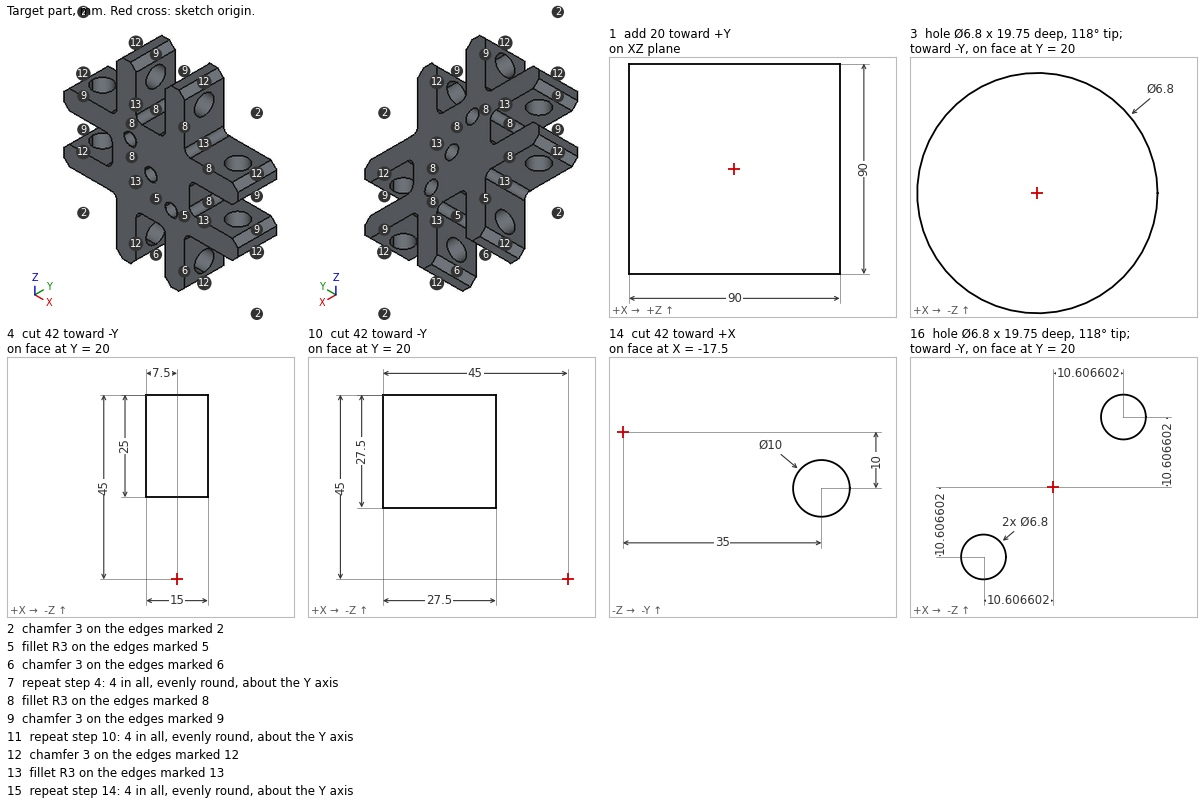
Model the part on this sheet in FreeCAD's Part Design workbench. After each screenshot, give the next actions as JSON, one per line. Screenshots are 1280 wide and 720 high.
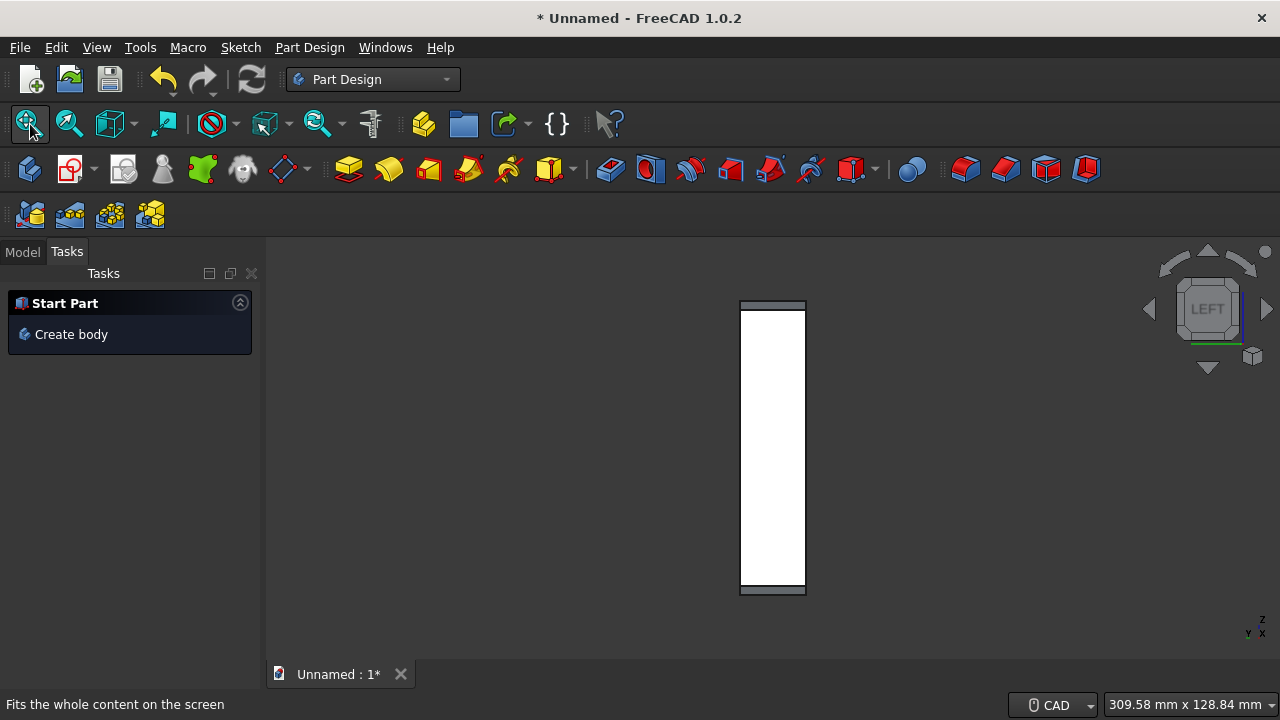
{"action": "key", "text": "v 3"}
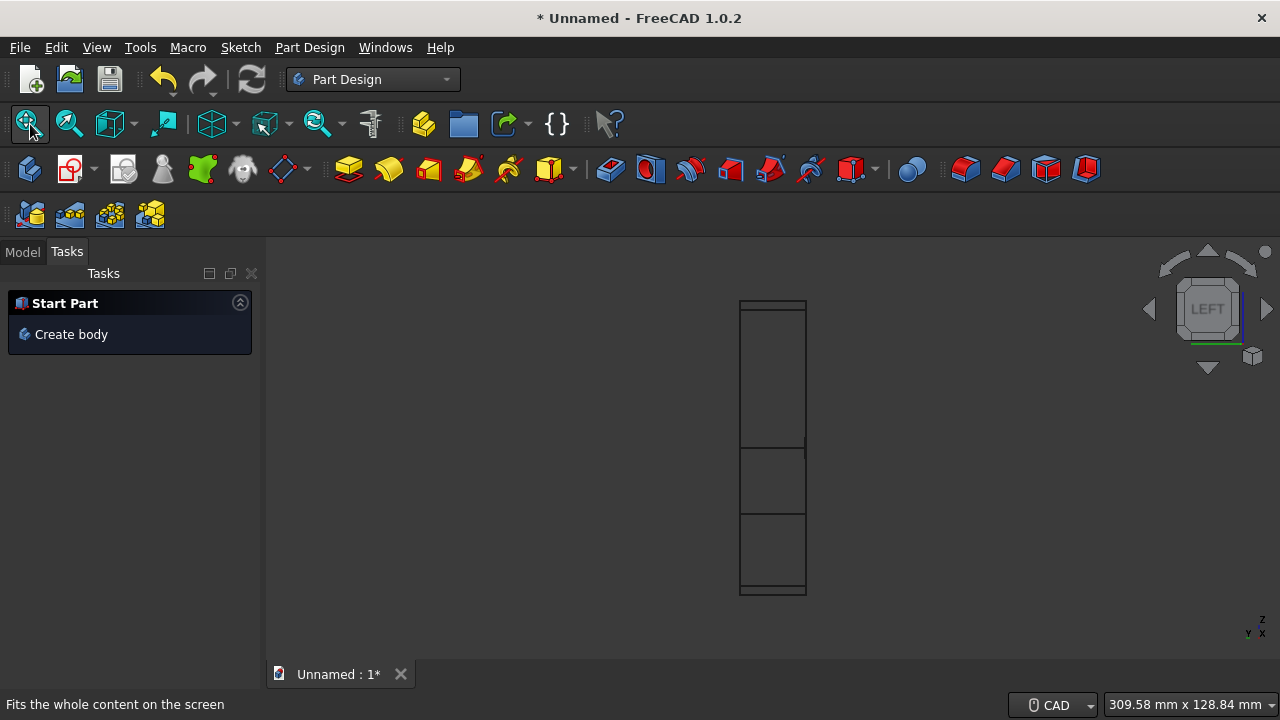
{"action": "key", "text": "0"}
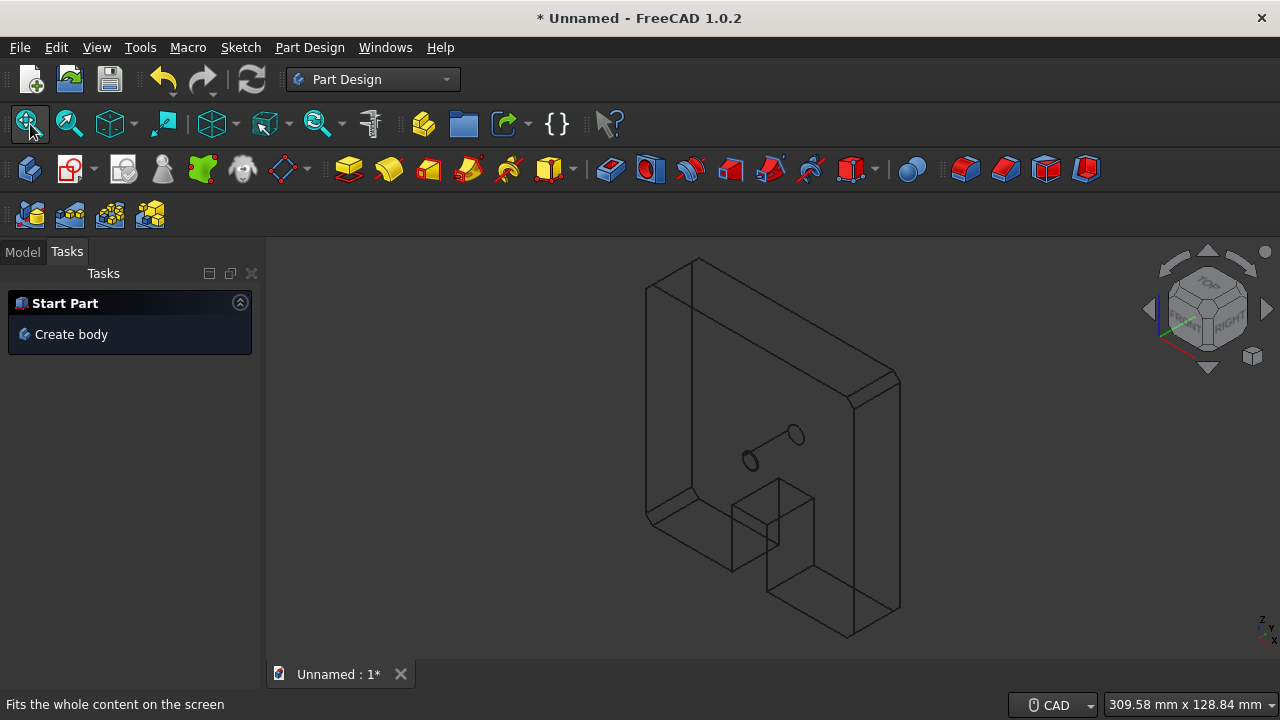
{"action": "left_click", "coordinate": [790, 511]}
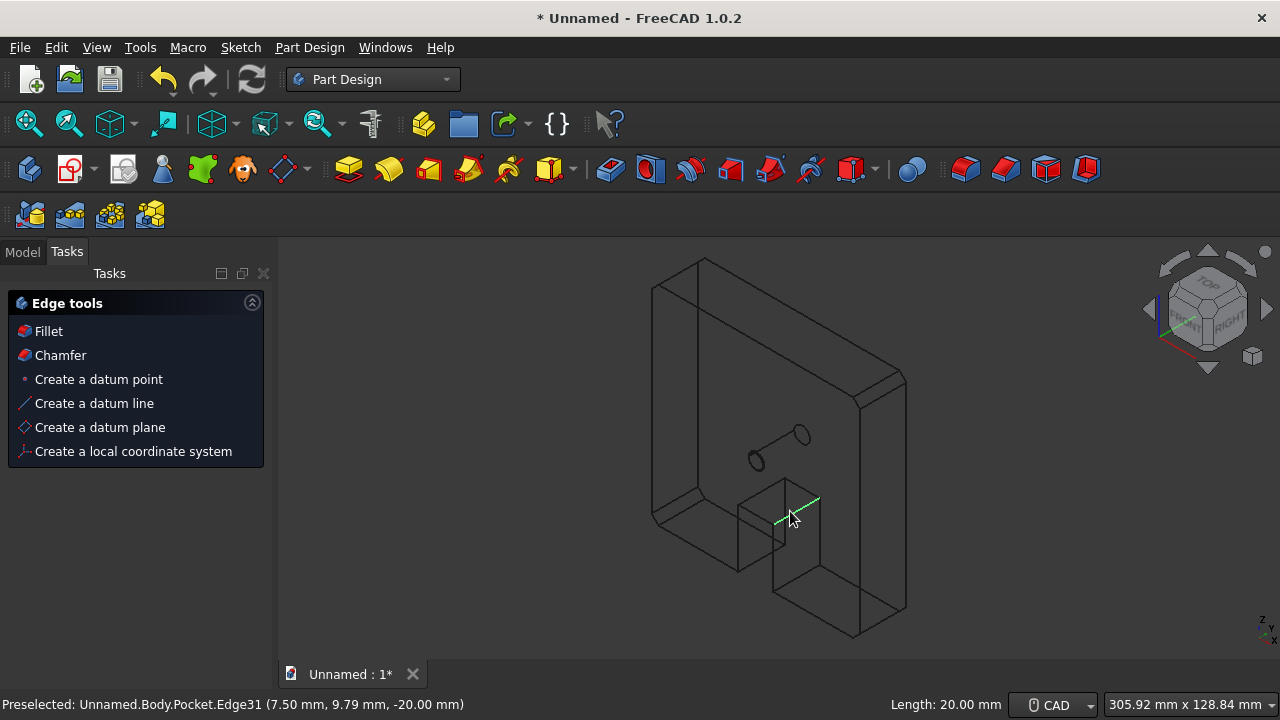
{"action": "left_click", "coordinate": [762, 490], "text": "ctrl"}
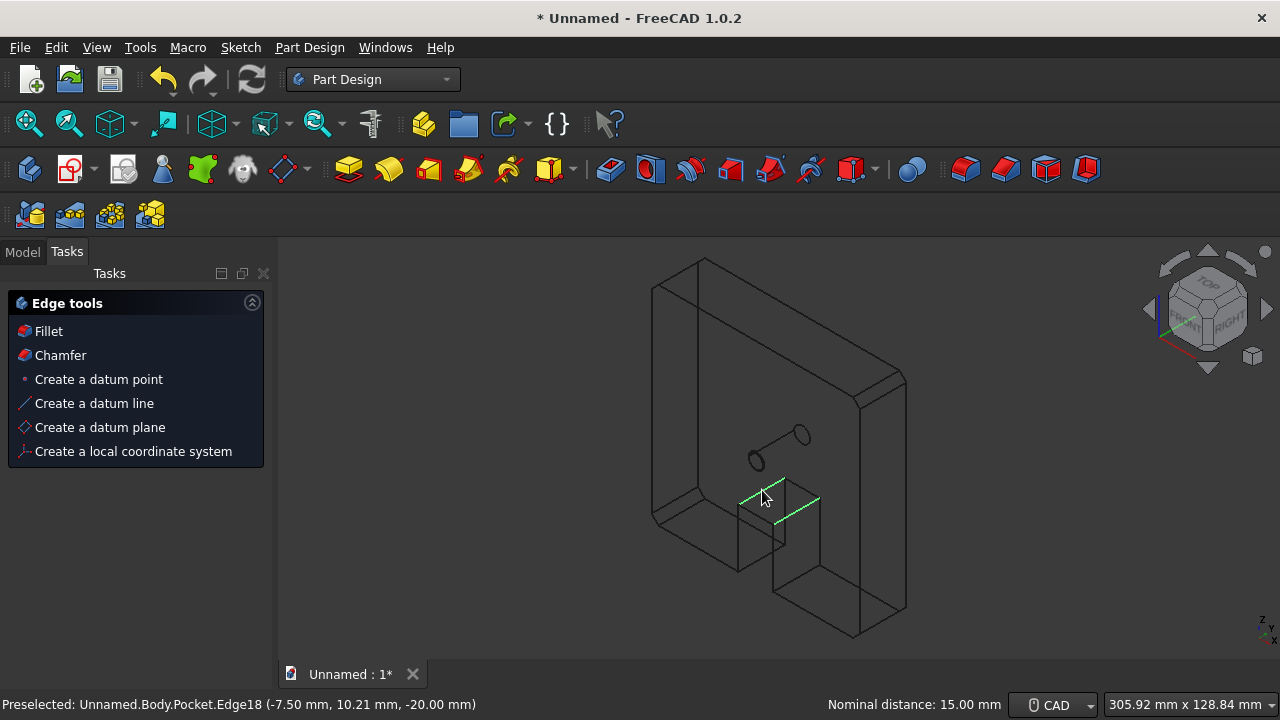
{"action": "key", "text": "v 1"}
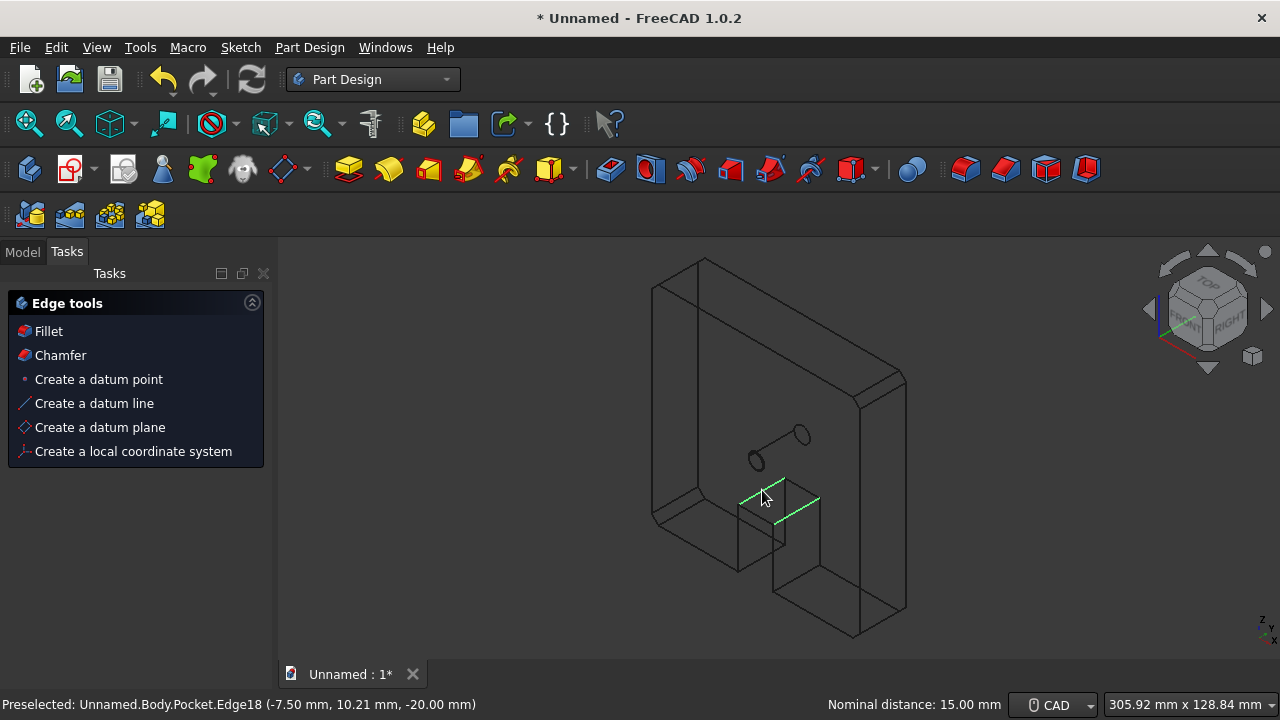
{"action": "left_click", "coordinate": [966, 170]}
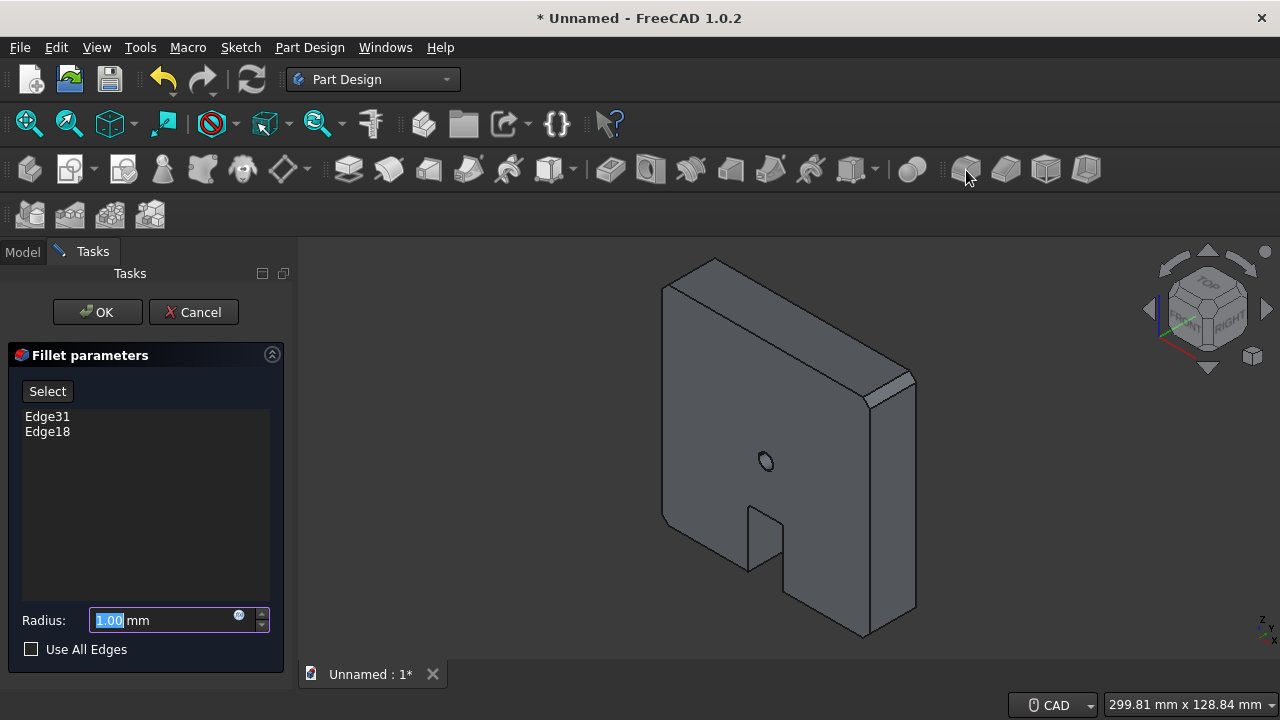
{"action": "type", "text": "3"}
{"action": "key", "text": "Tab"}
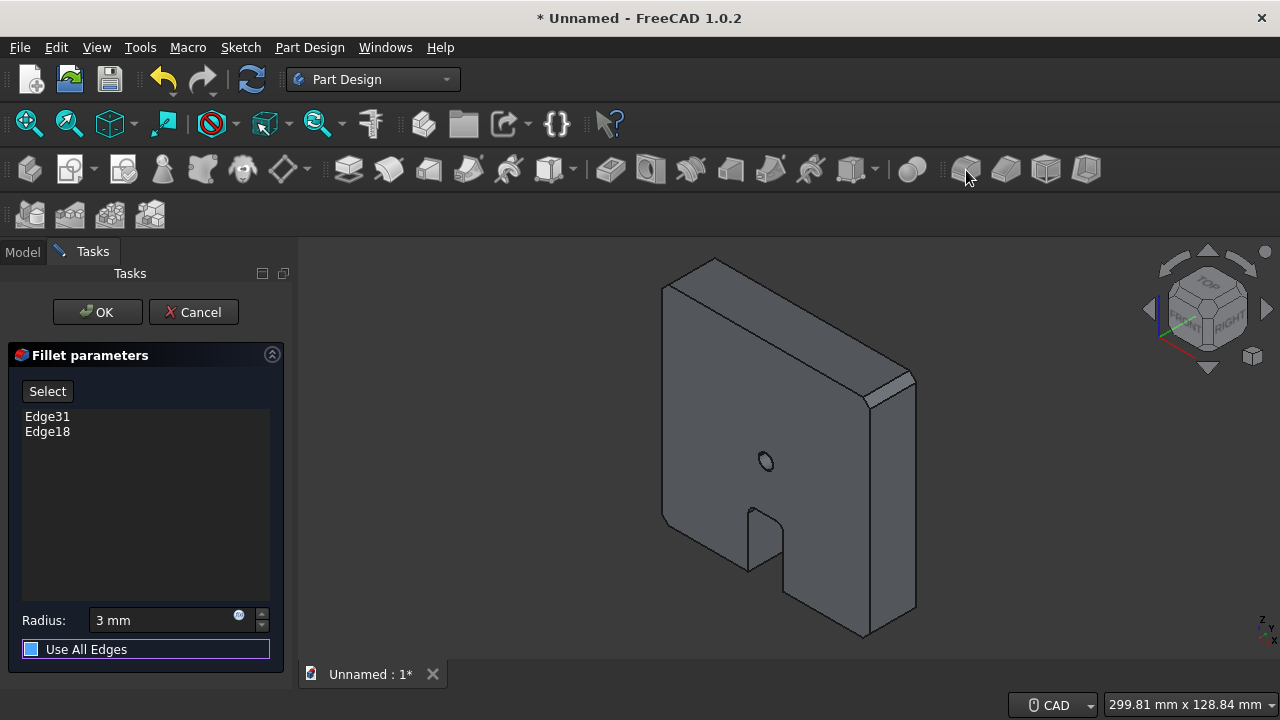
{"action": "left_click", "coordinate": [98, 312]}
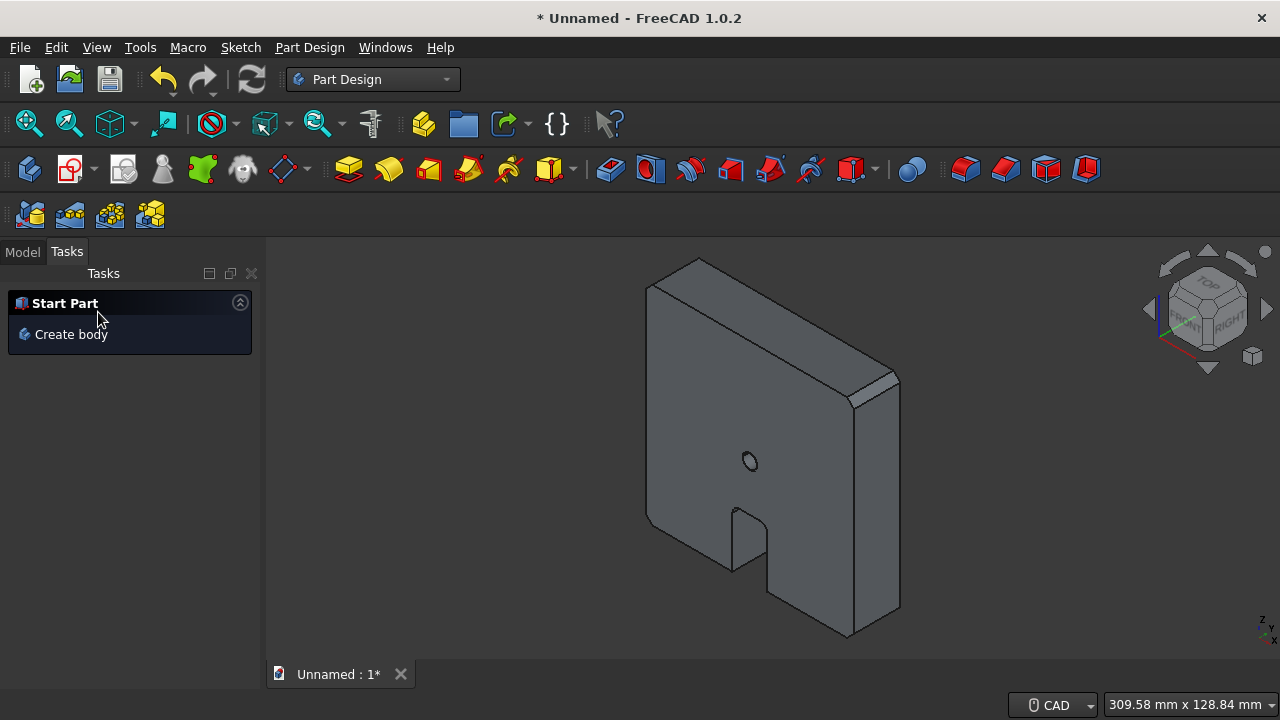
{"action": "key", "text": "2"}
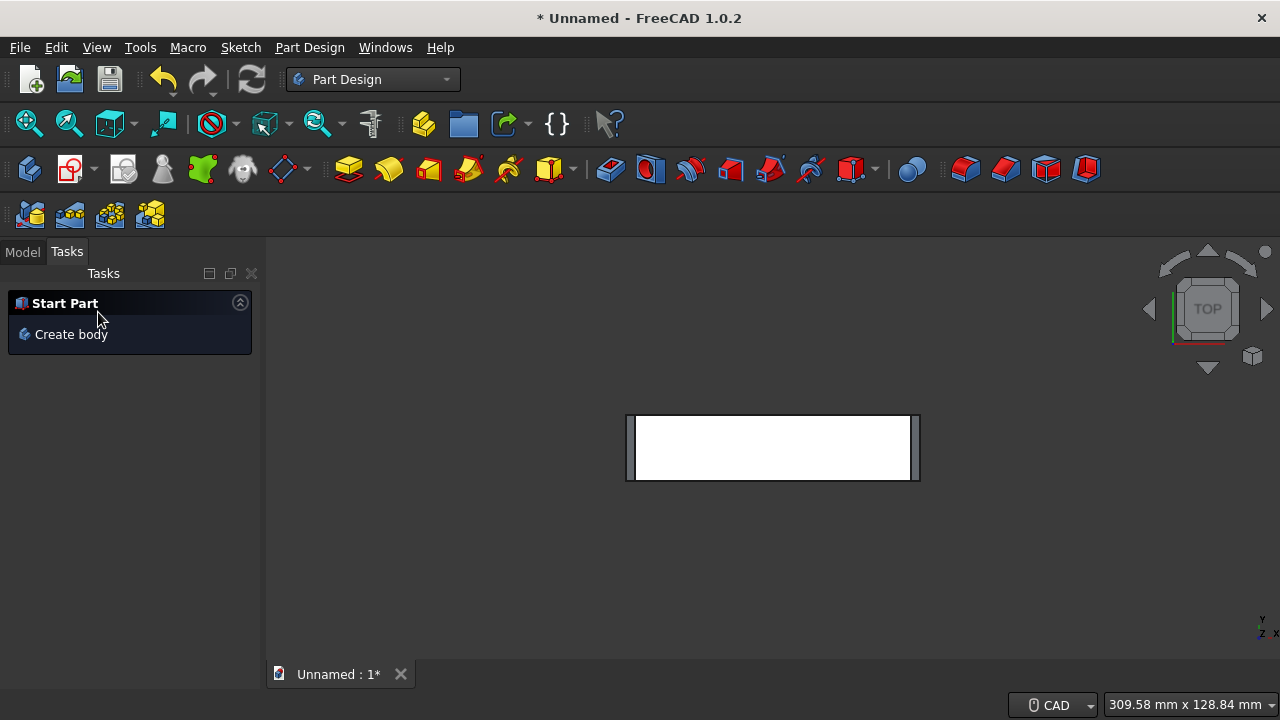
{"action": "left_click", "coordinate": [30, 124]}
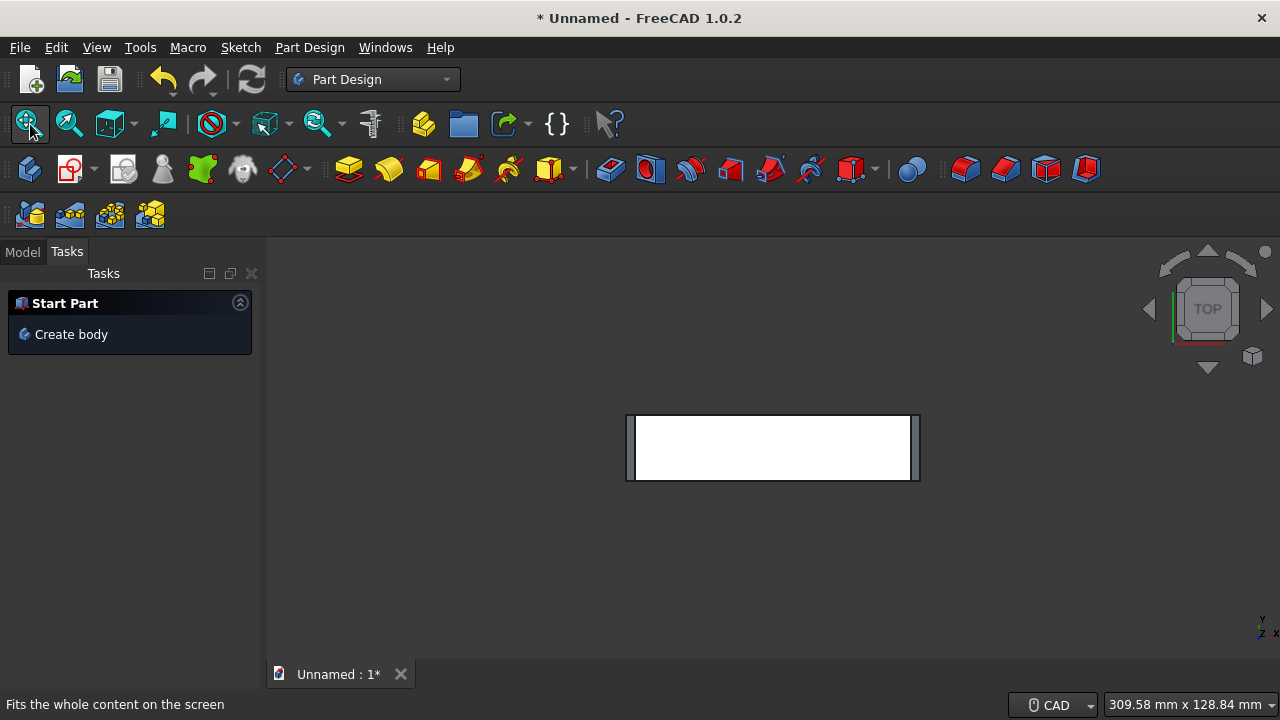
{"action": "key", "text": "0"}